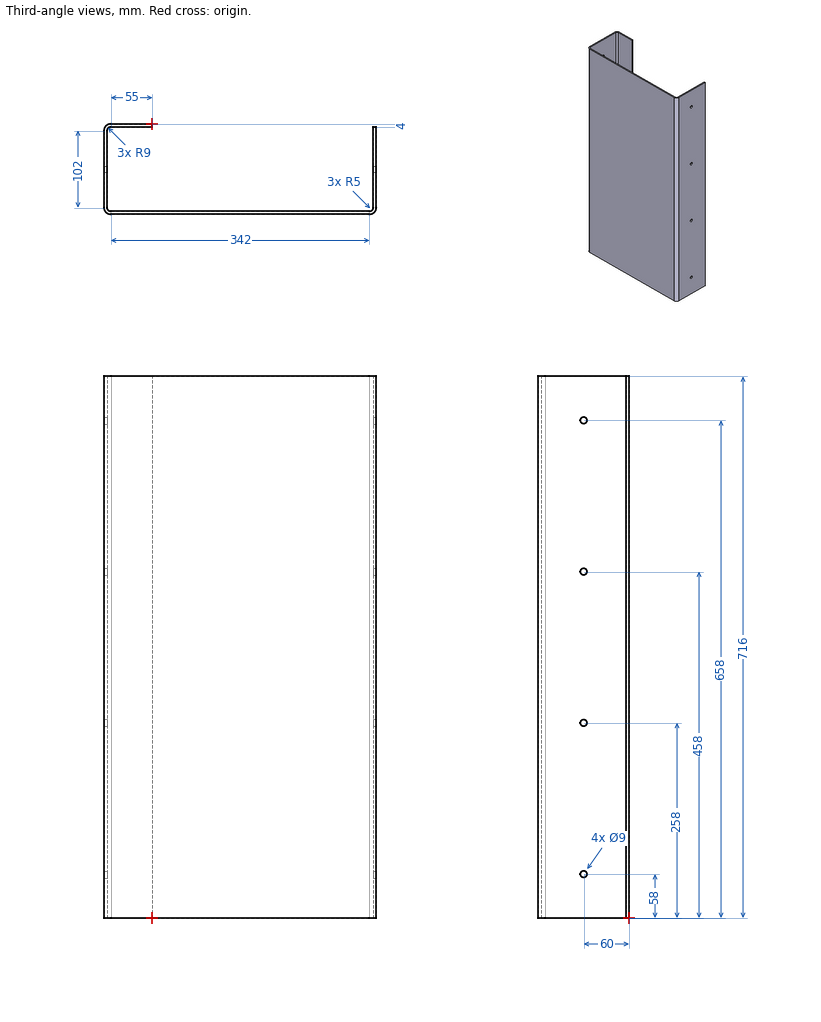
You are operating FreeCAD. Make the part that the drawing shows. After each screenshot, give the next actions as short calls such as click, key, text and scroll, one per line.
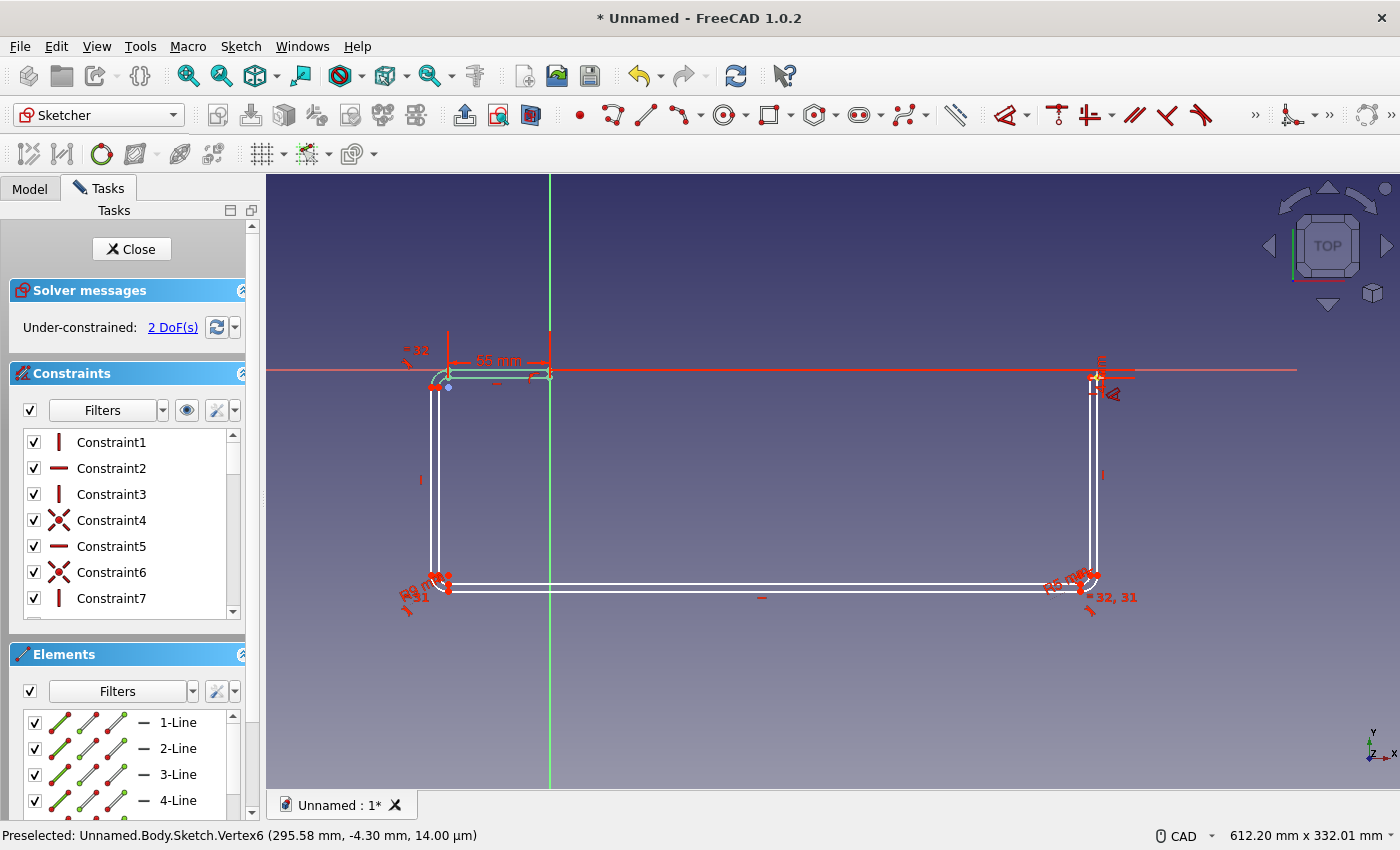
scroll(431, 444, up, 4)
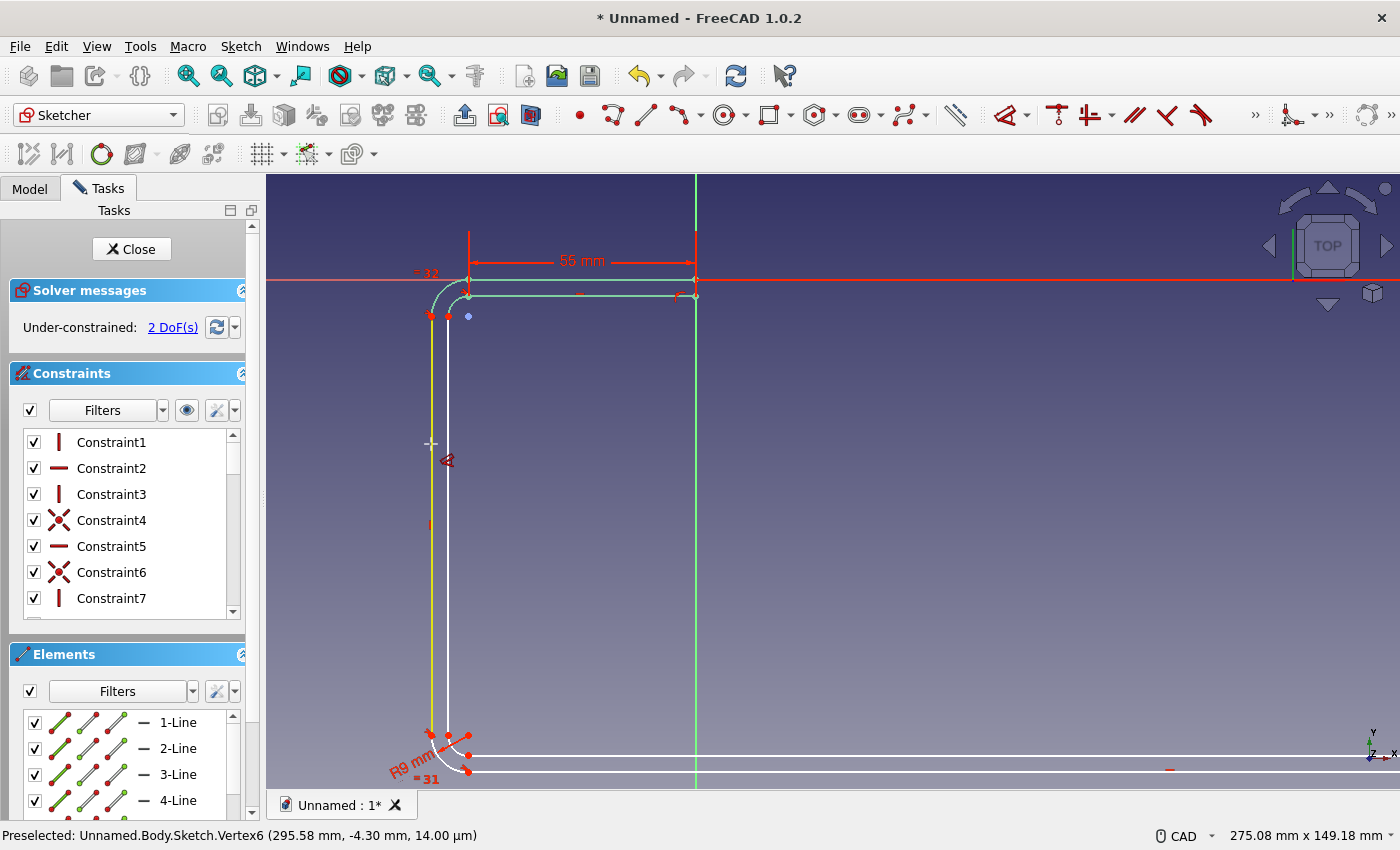
click(432, 442)
click(398, 526)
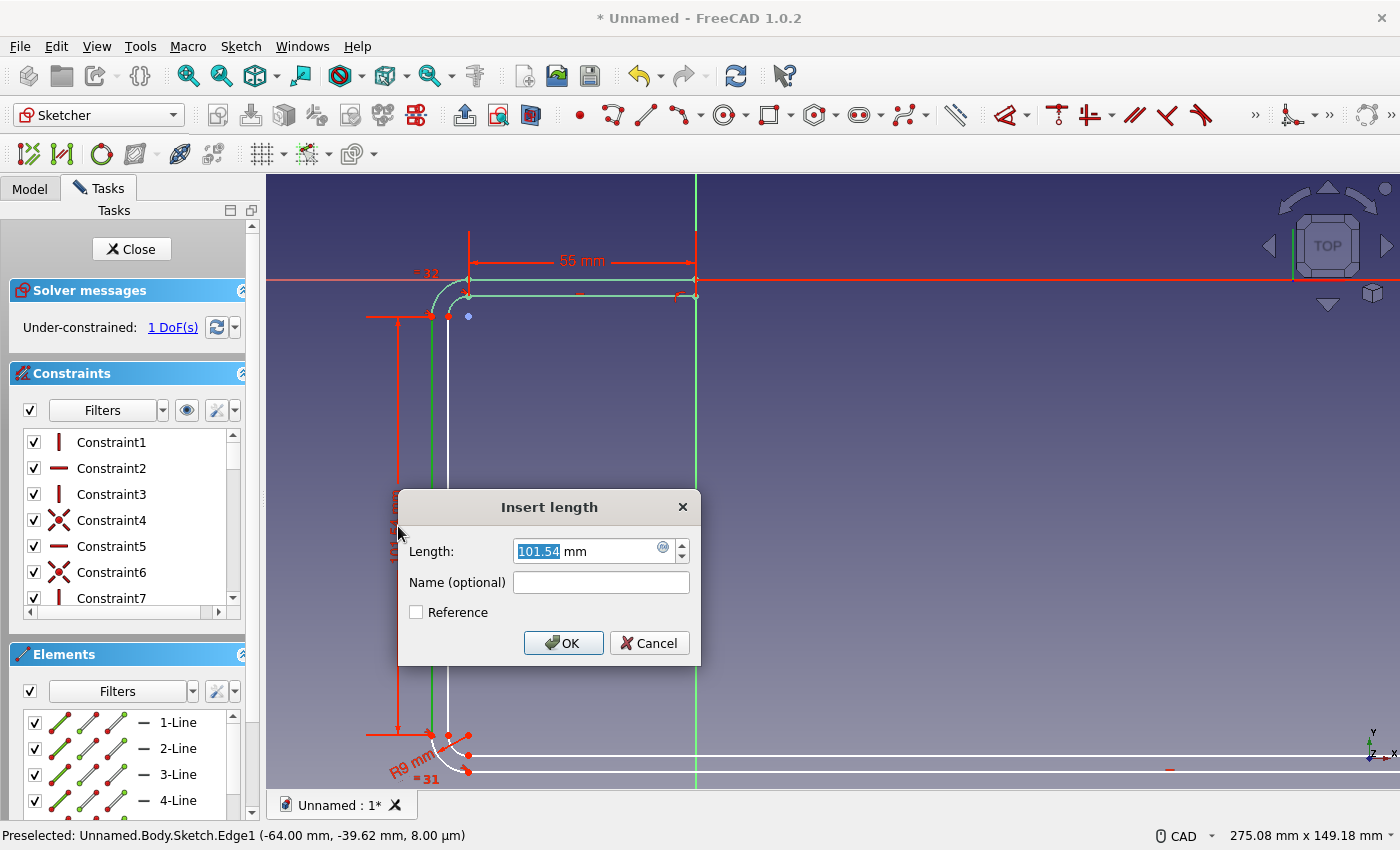
text(102)
key(Return)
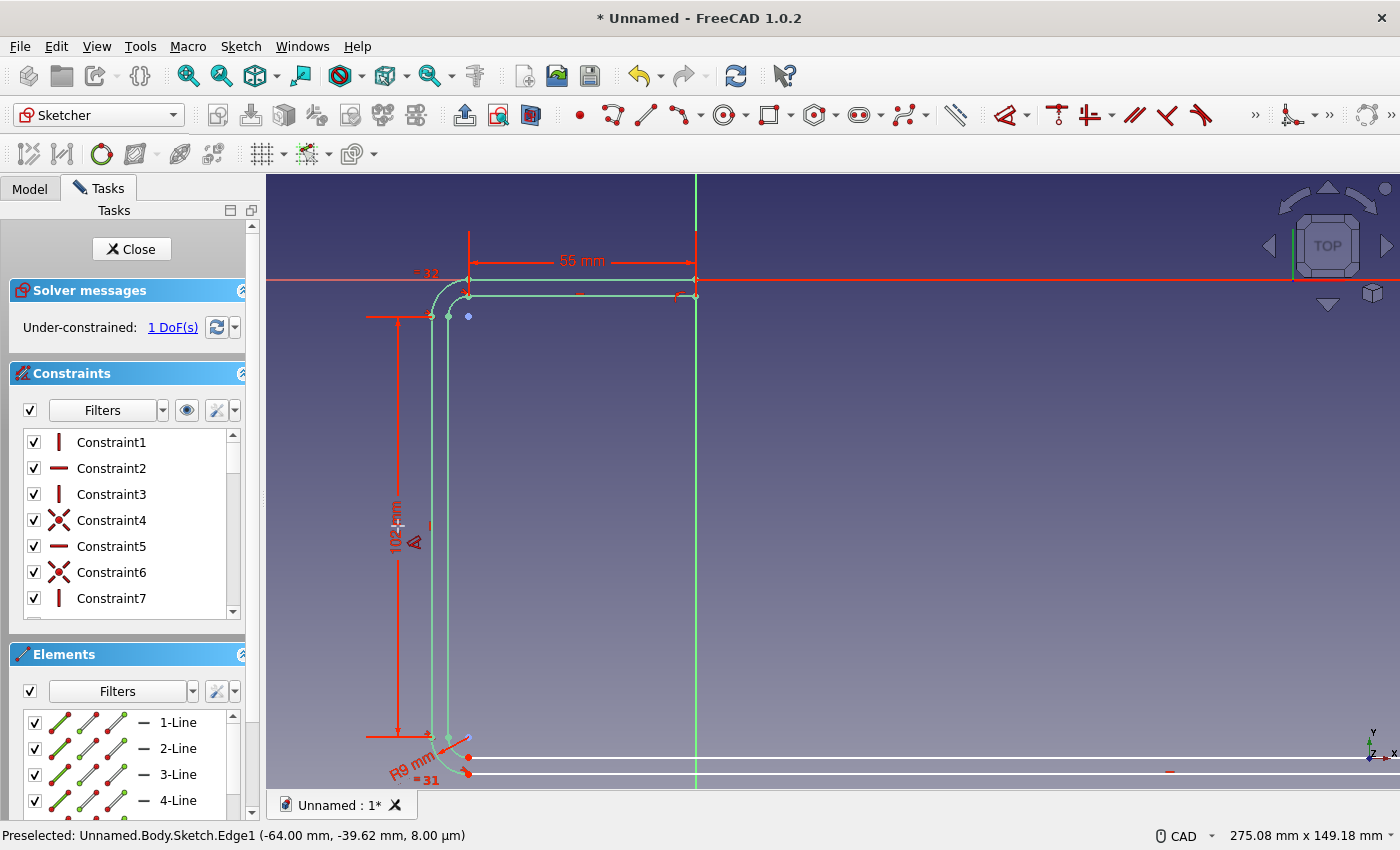
scroll(431, 444, down, 4)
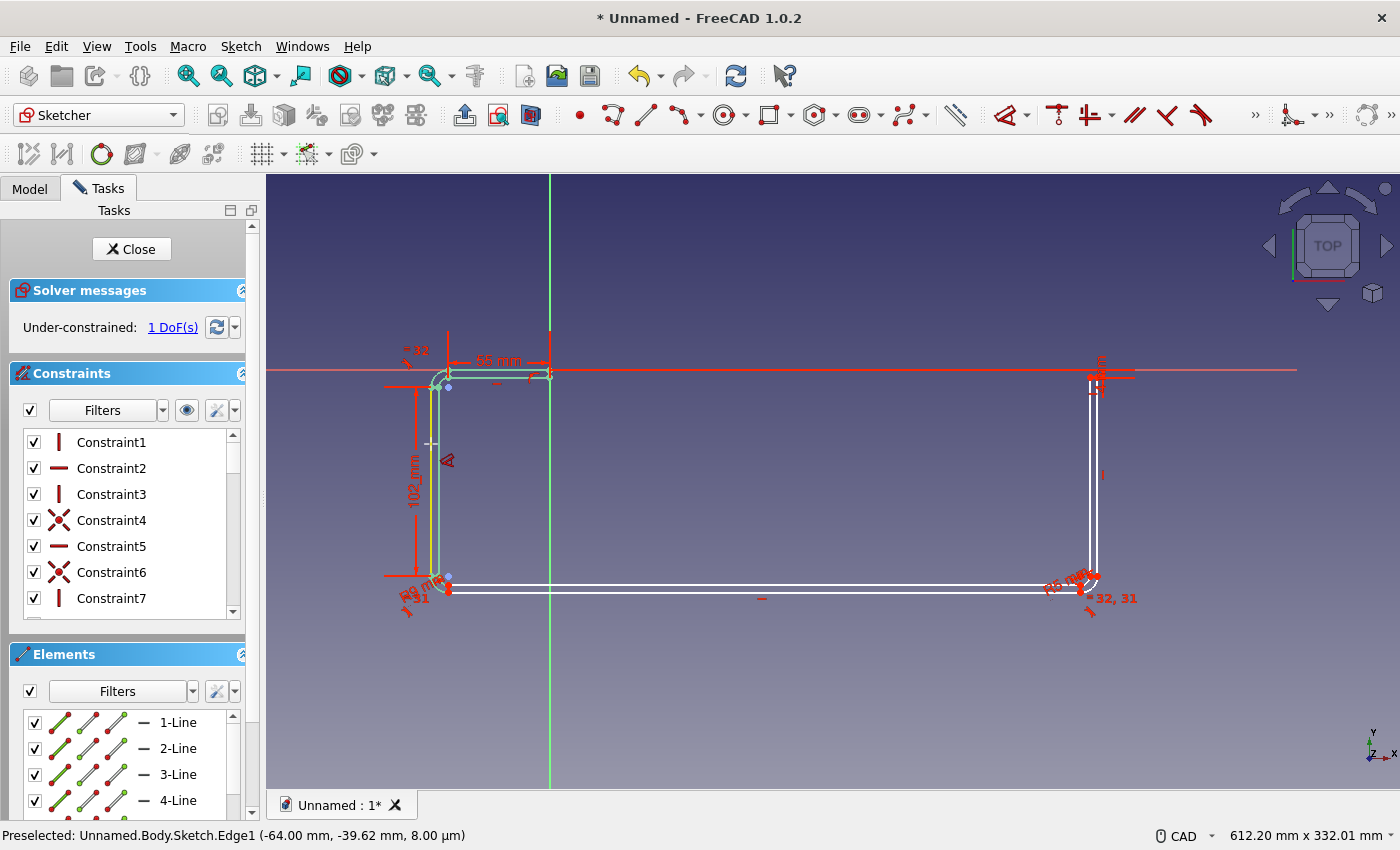
scroll(638, 593, up, 4)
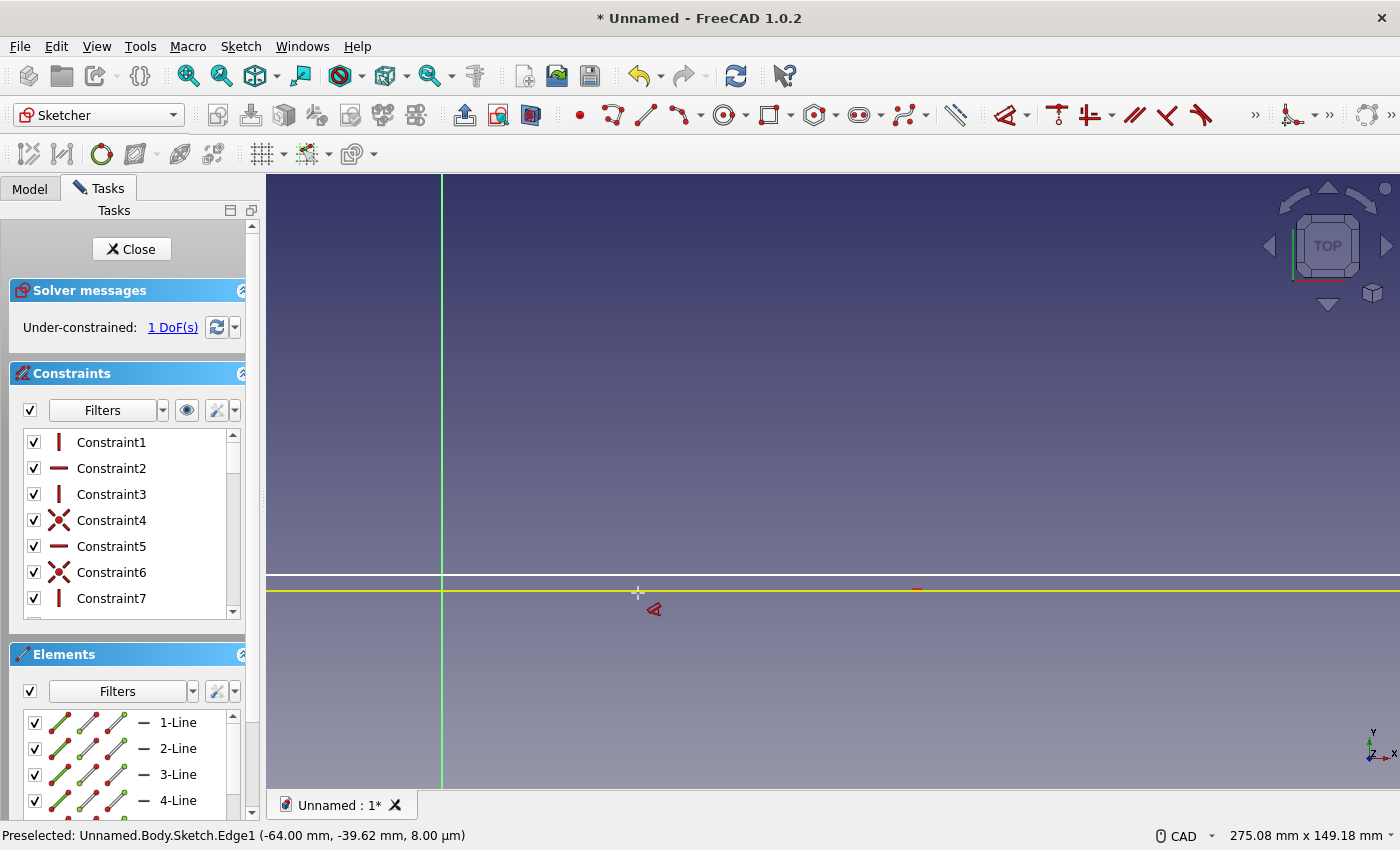
click(637, 591)
click(764, 625)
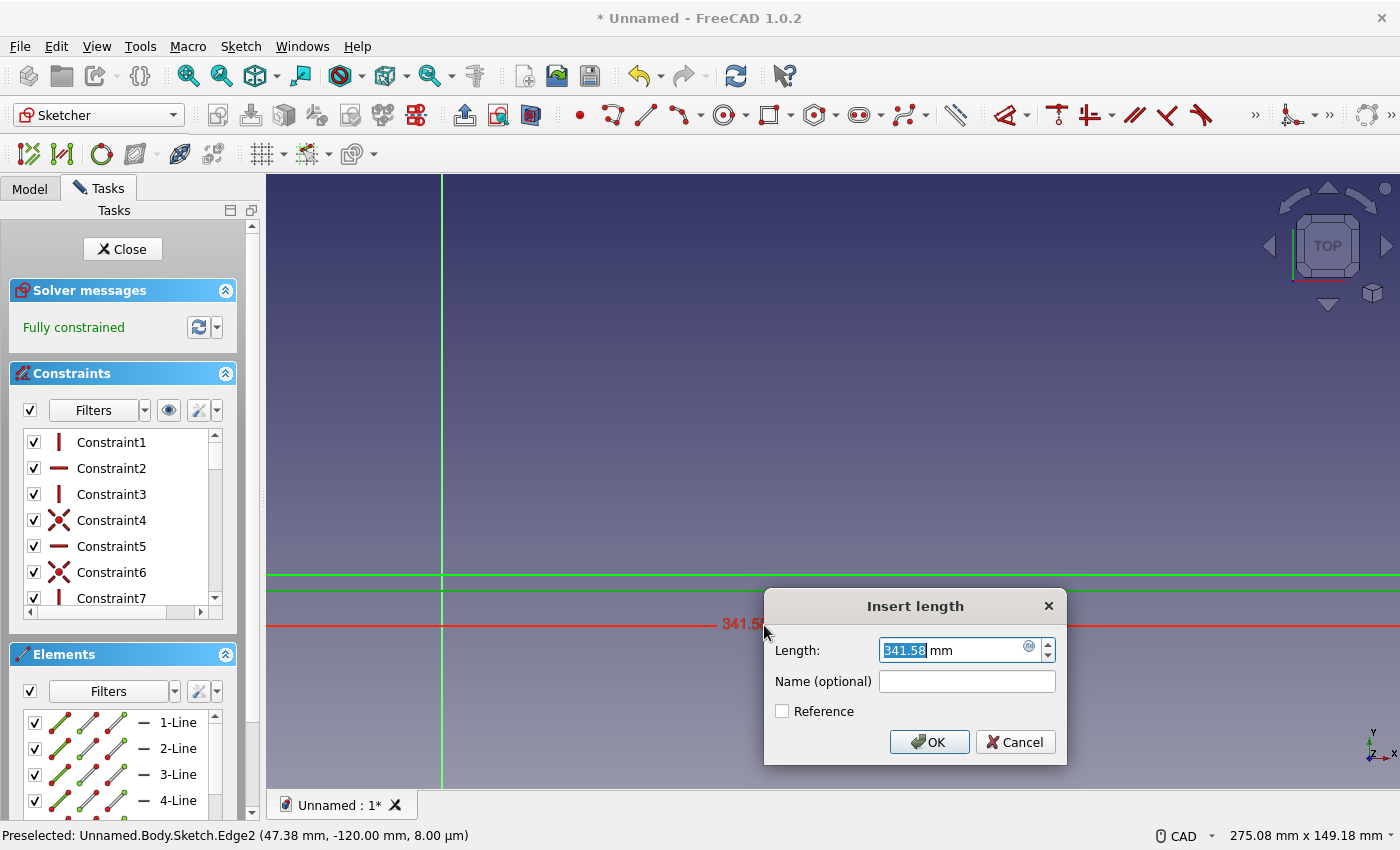
text(342)
key(Return)
key(Escape)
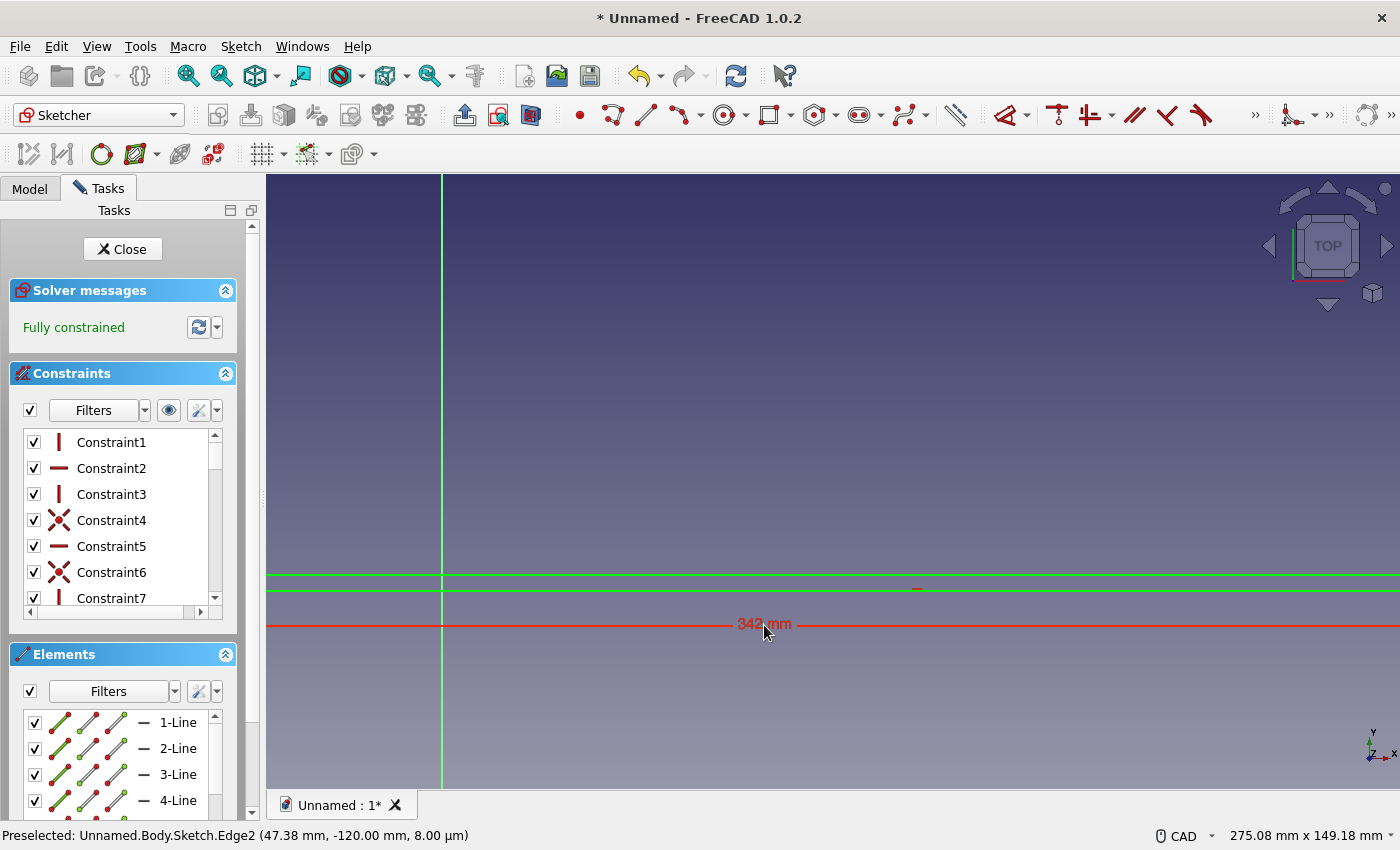
click(123, 249)